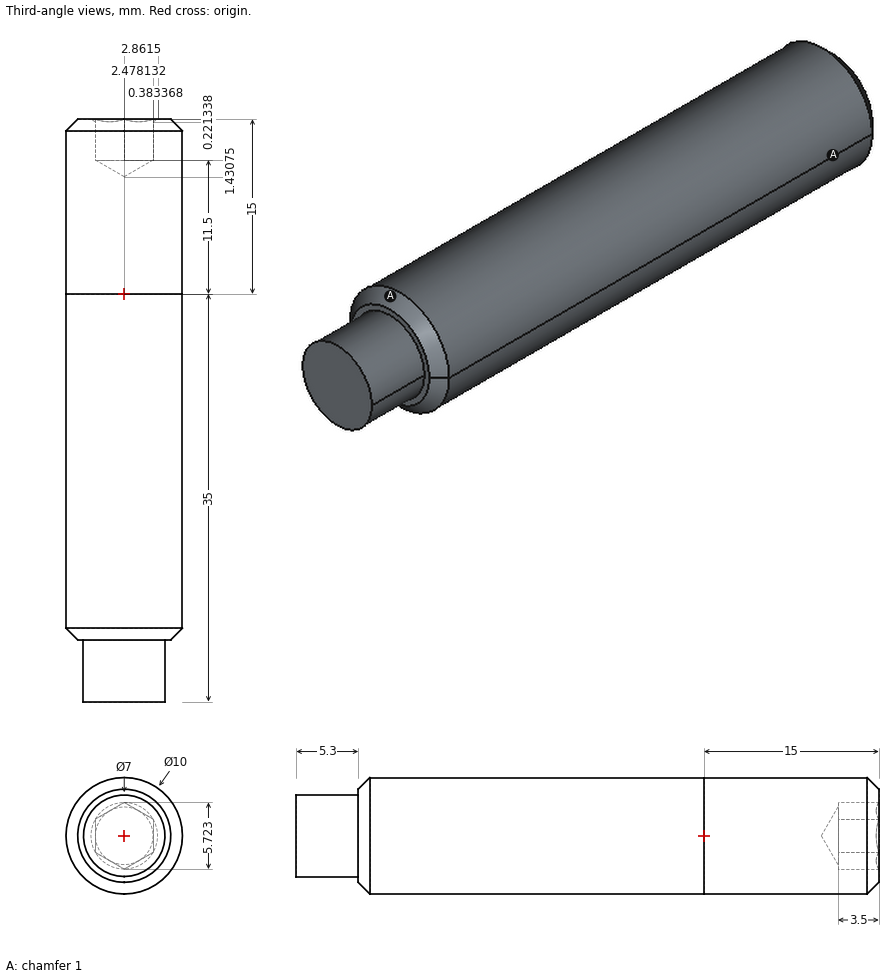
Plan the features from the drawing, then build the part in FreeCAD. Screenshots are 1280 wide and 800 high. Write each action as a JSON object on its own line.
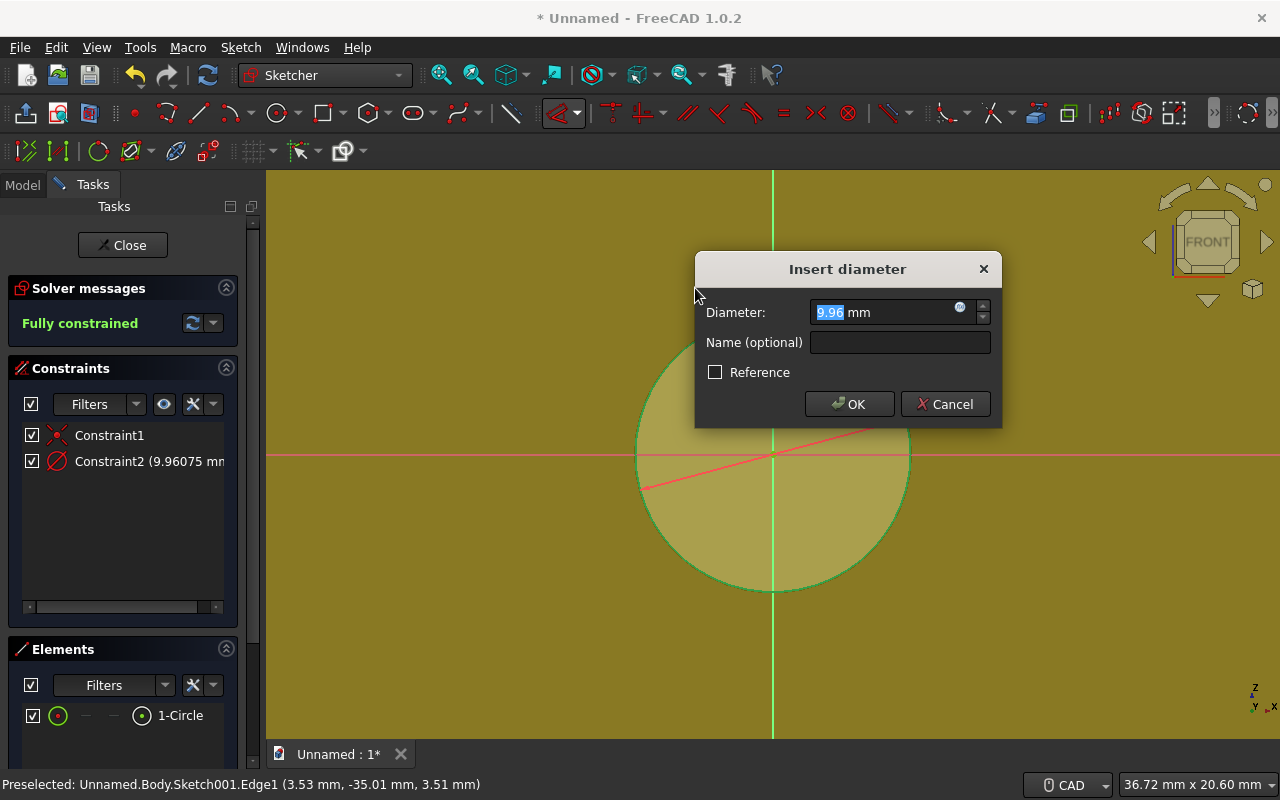
{"action": "type", "text": "10"}
{"action": "key", "text": "Return"}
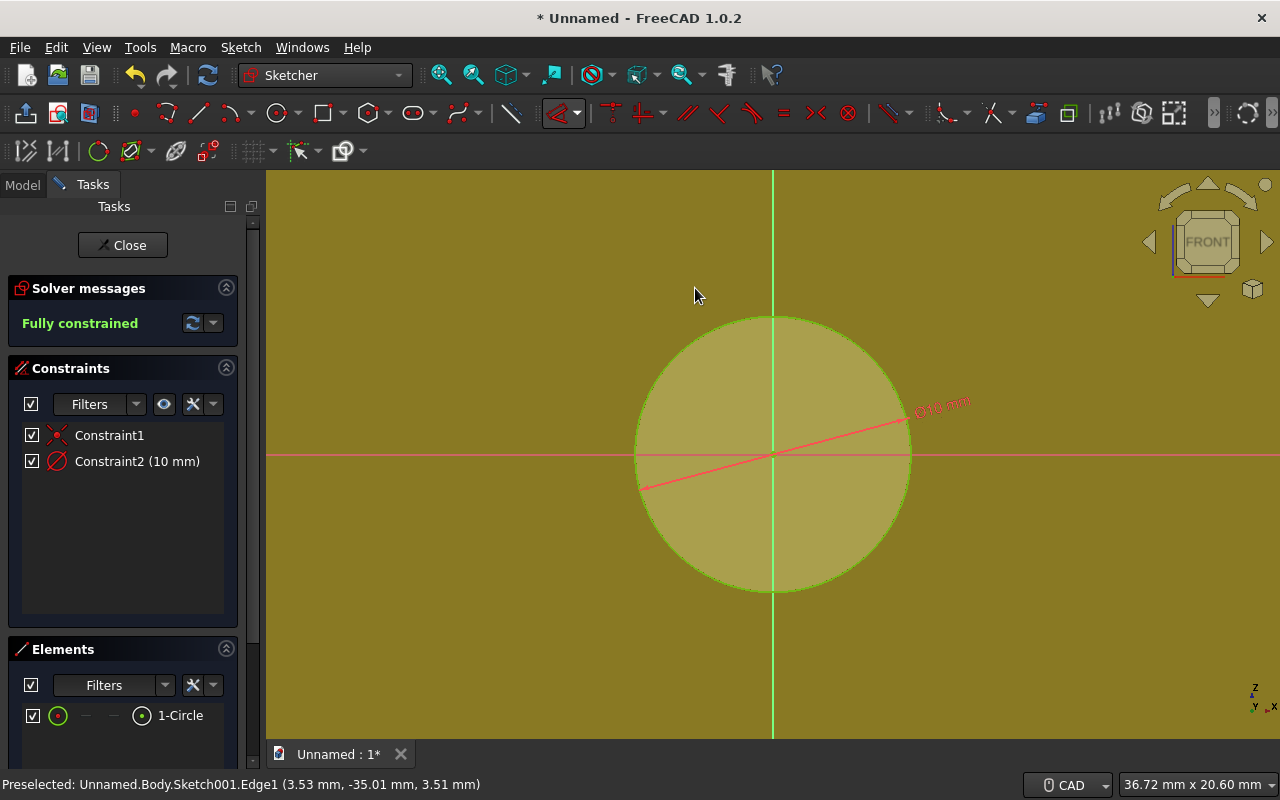
{"action": "left_click", "coordinate": [123, 245]}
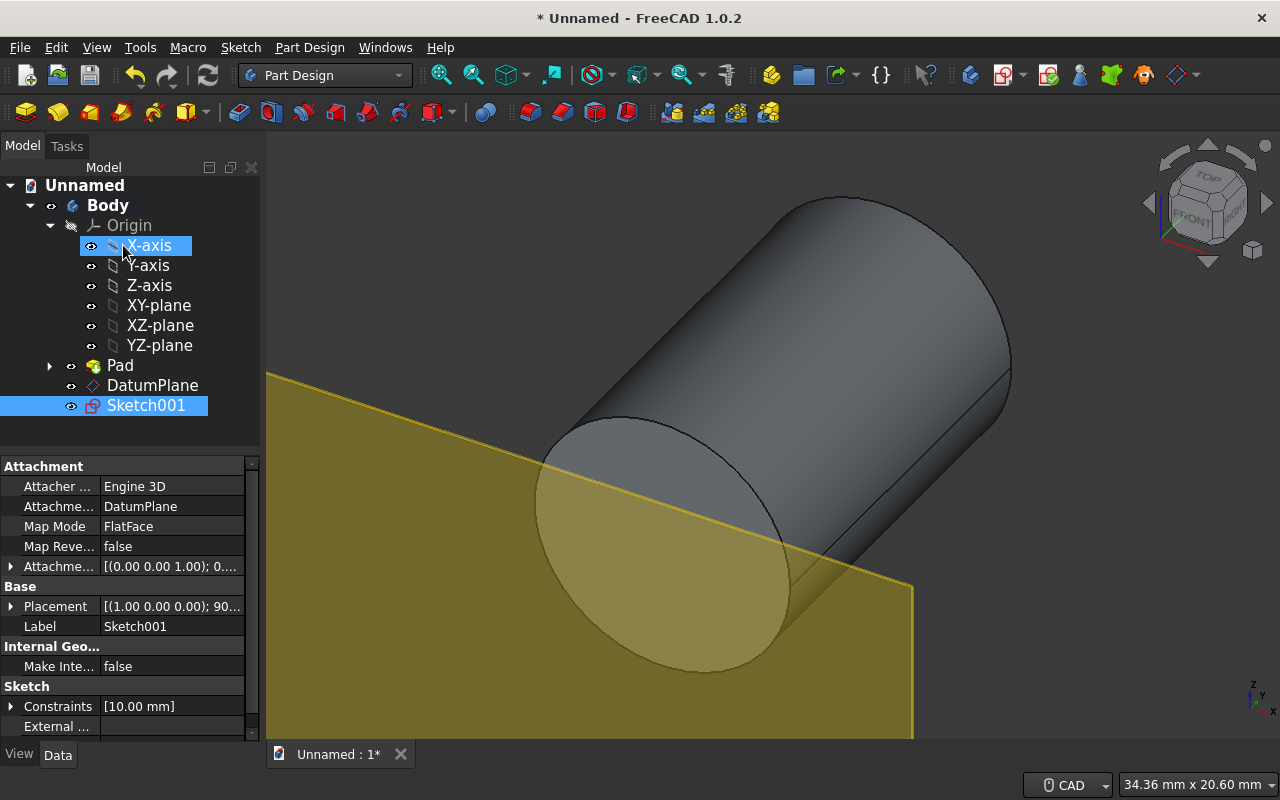
{"action": "left_click", "coordinate": [26, 112]}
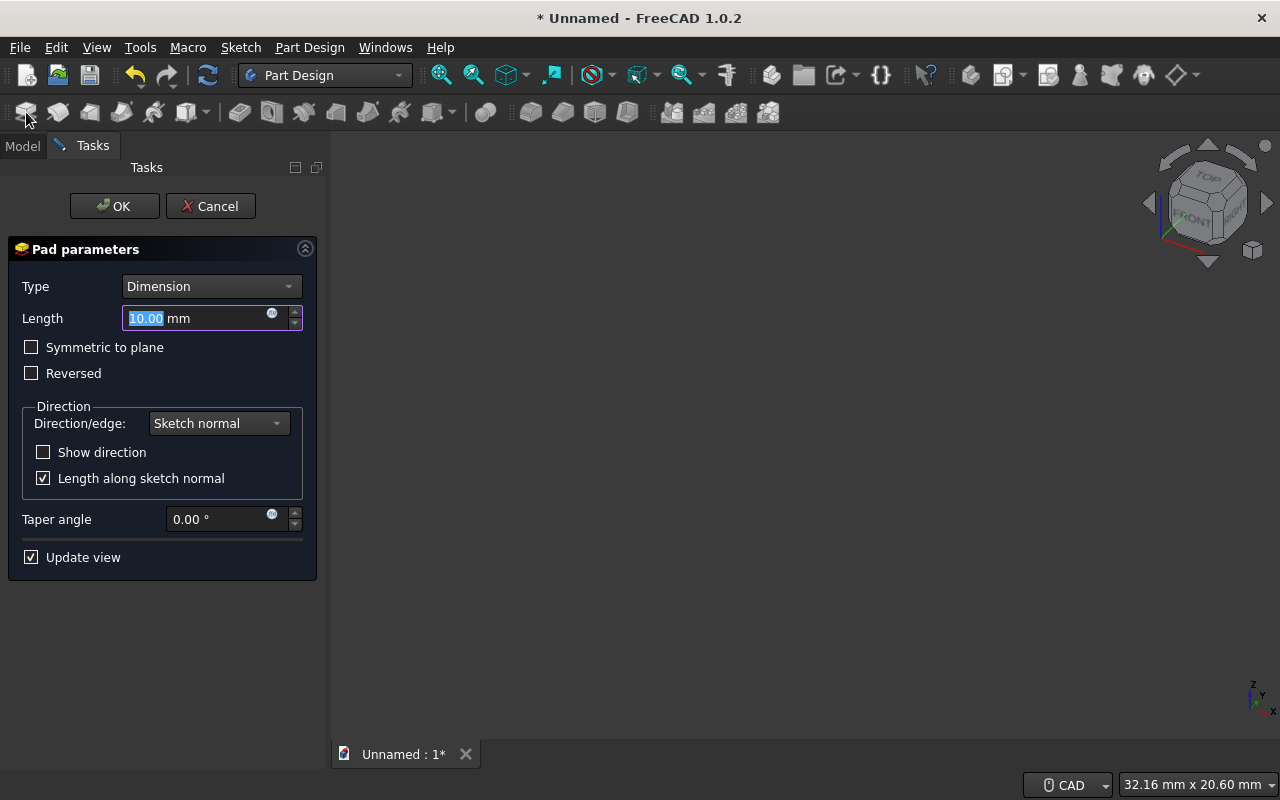
{"action": "type", "text": "35"}
{"action": "key", "text": "Tab"}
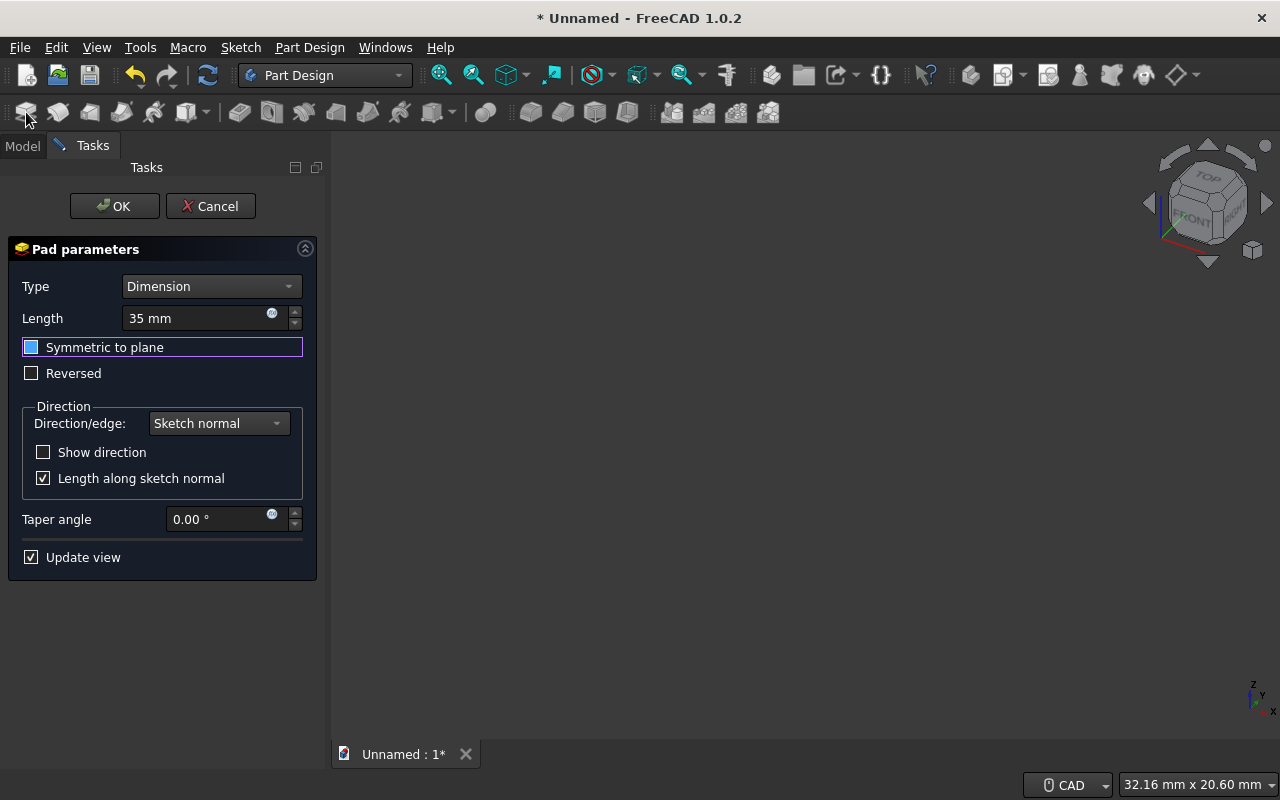
{"action": "left_click", "coordinate": [30, 373]}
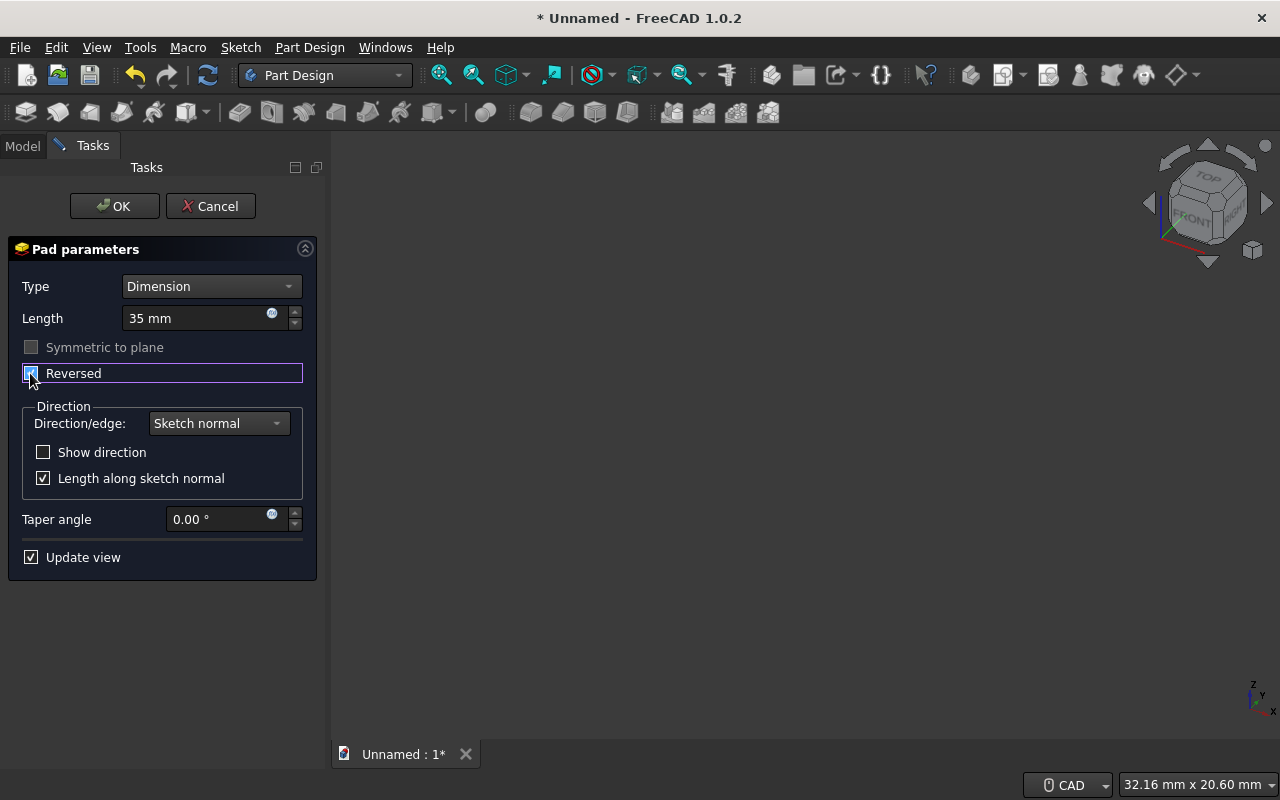
{"action": "left_click", "coordinate": [115, 206]}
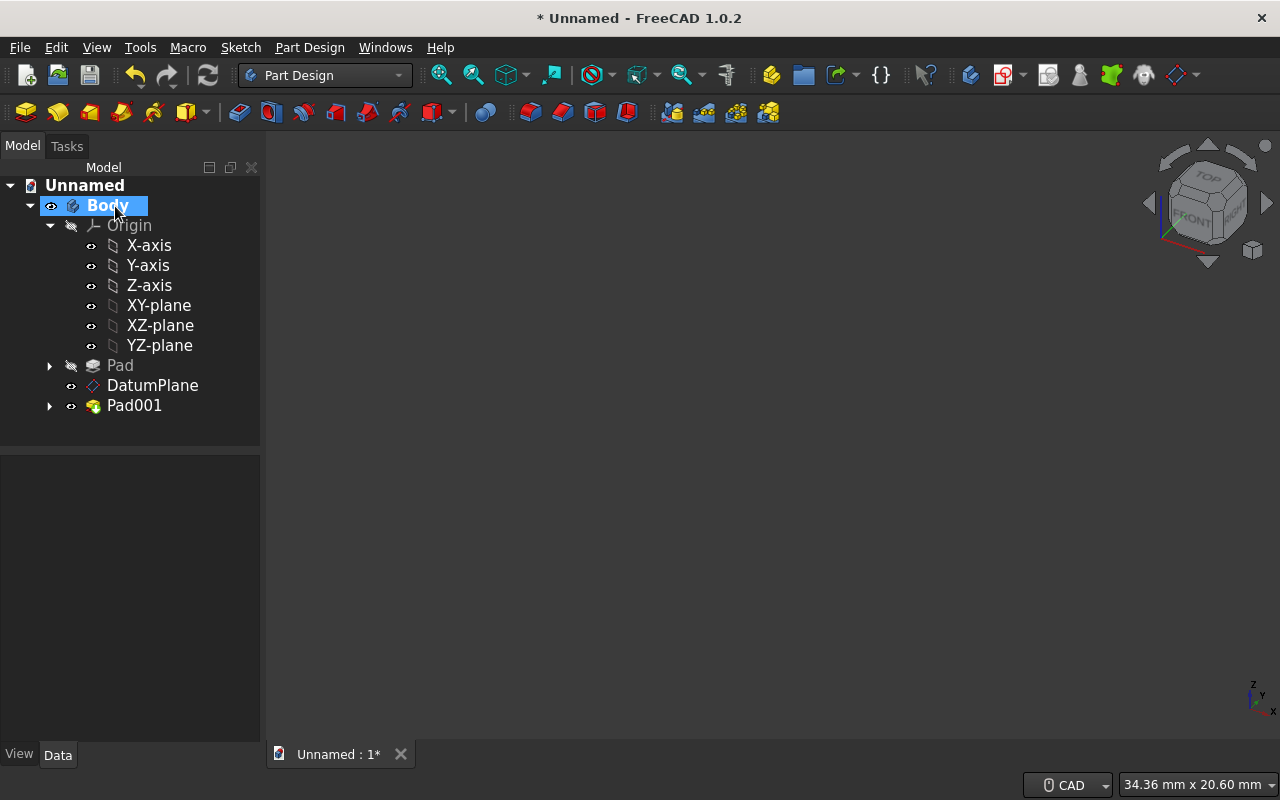
{"action": "left_click", "coordinate": [116, 386]}
{"action": "key", "text": "space"}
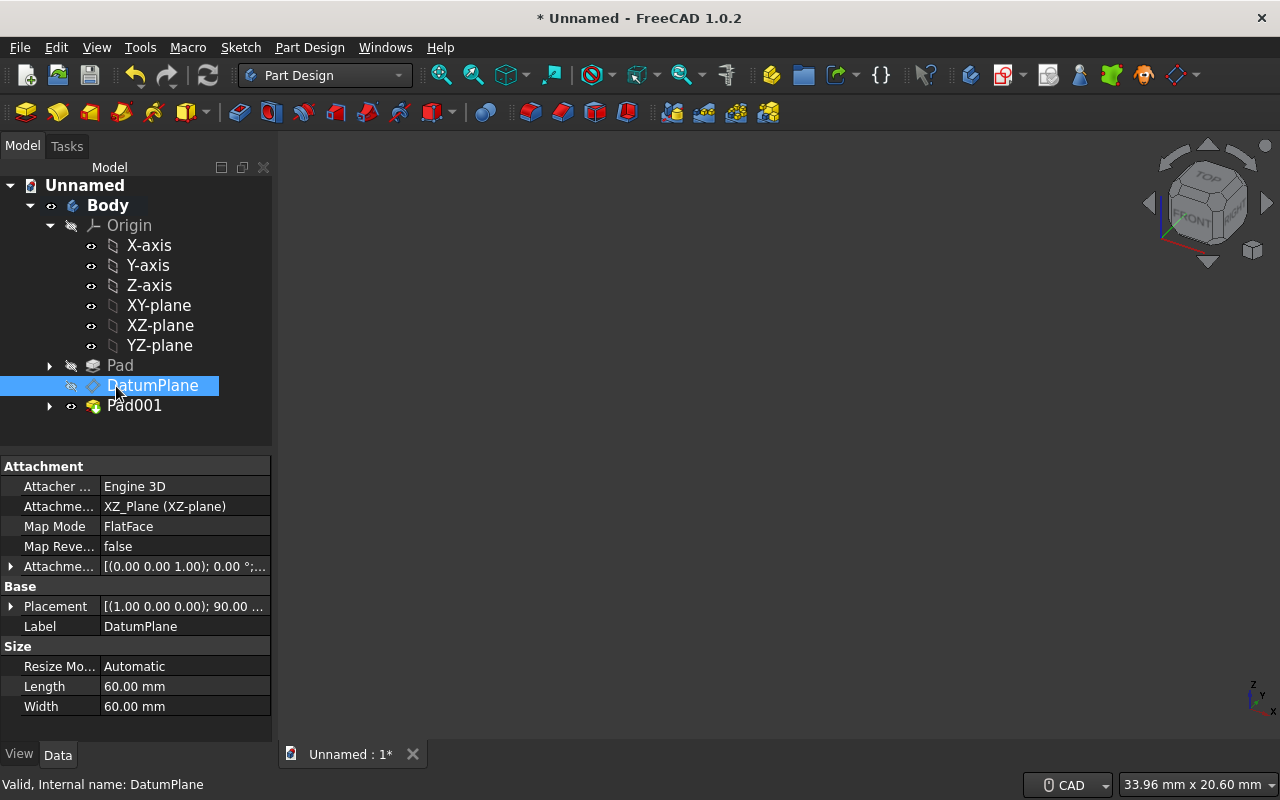
{"action": "left_click", "coordinate": [442, 76]}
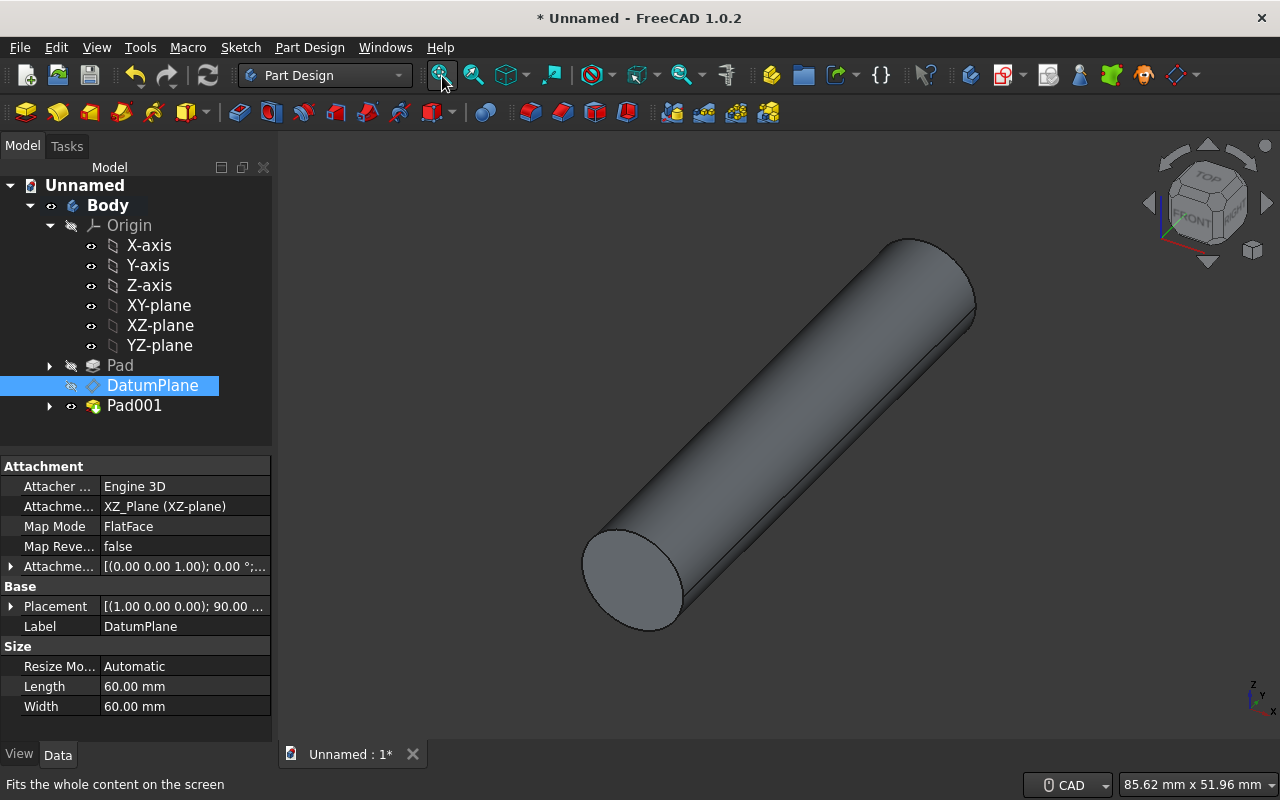
{"action": "key", "text": "4"}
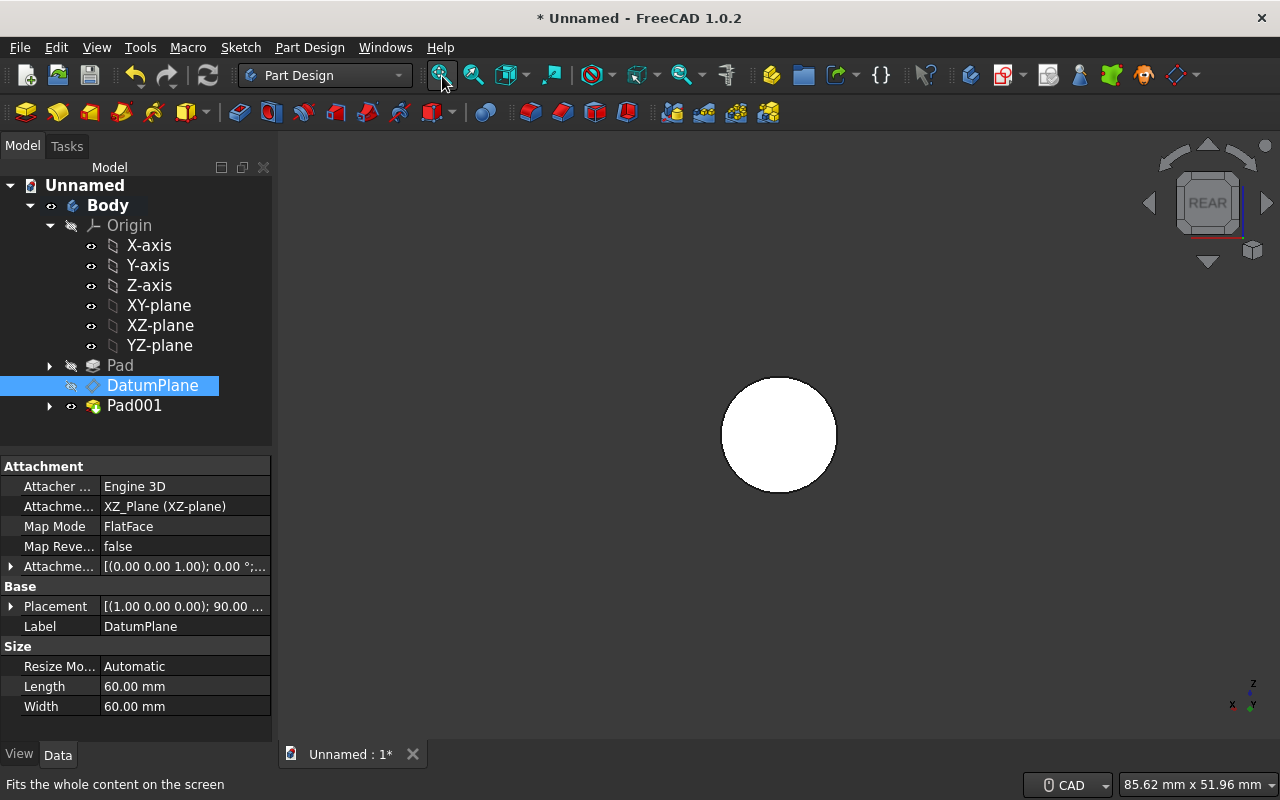
{"action": "left_click", "coordinate": [442, 76]}